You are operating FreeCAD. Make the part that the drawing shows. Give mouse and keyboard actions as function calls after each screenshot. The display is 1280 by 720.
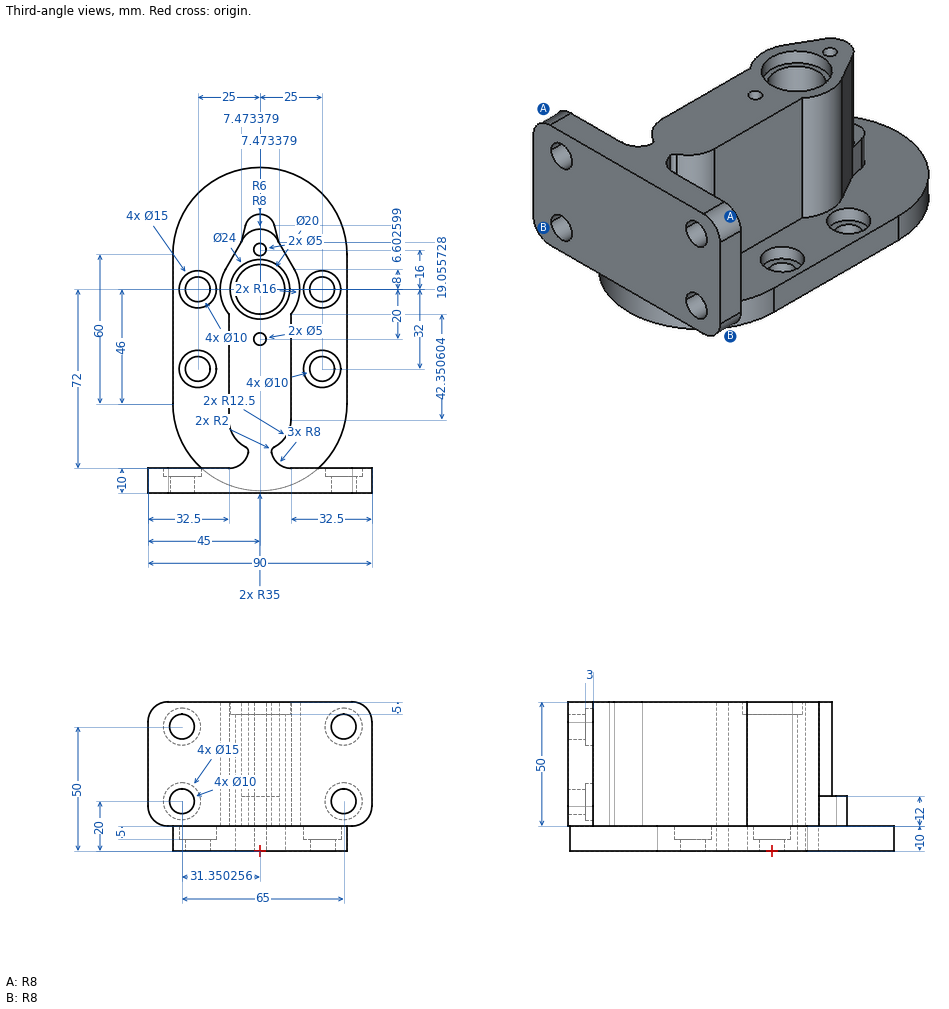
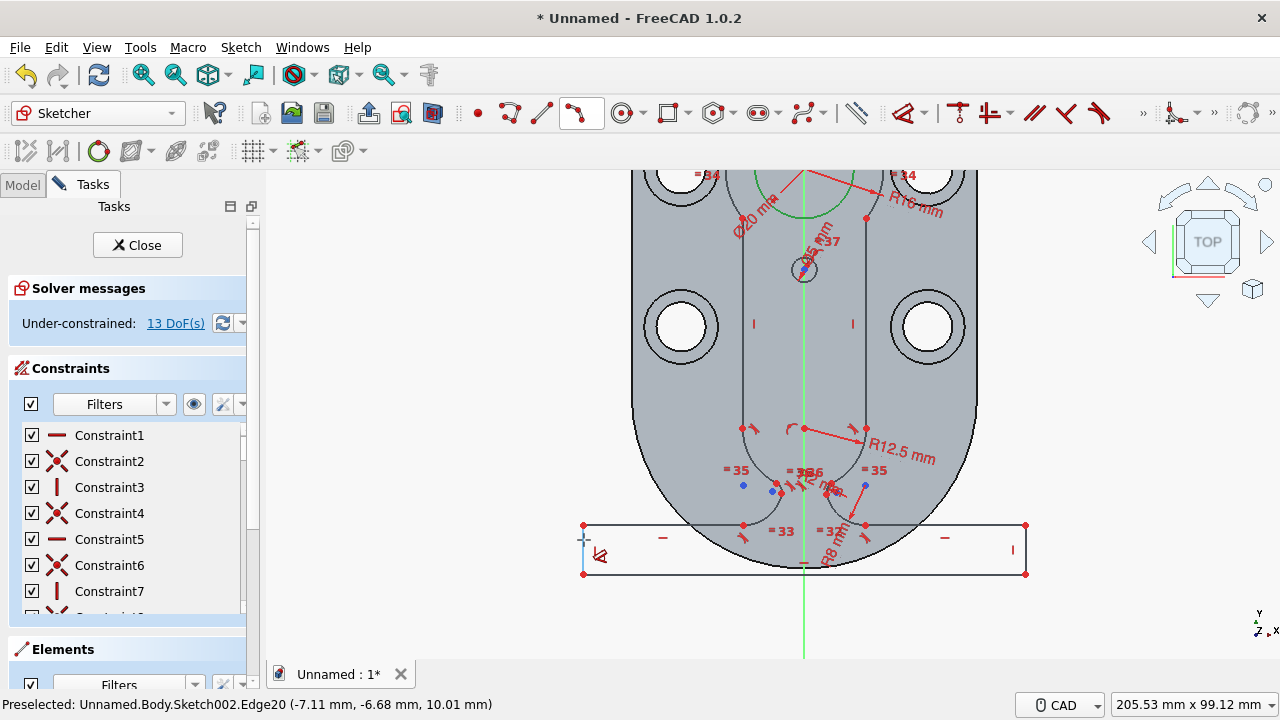
click(583, 540)
click(549, 550)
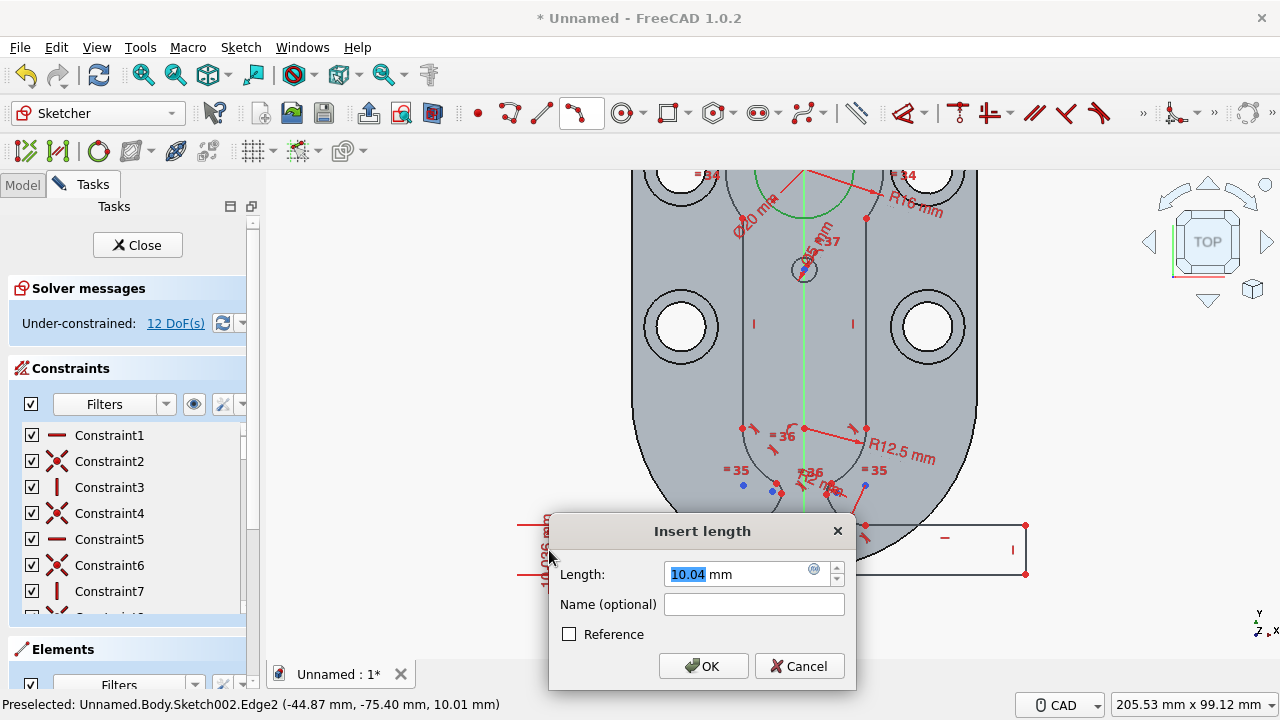
text(10)
key(Return)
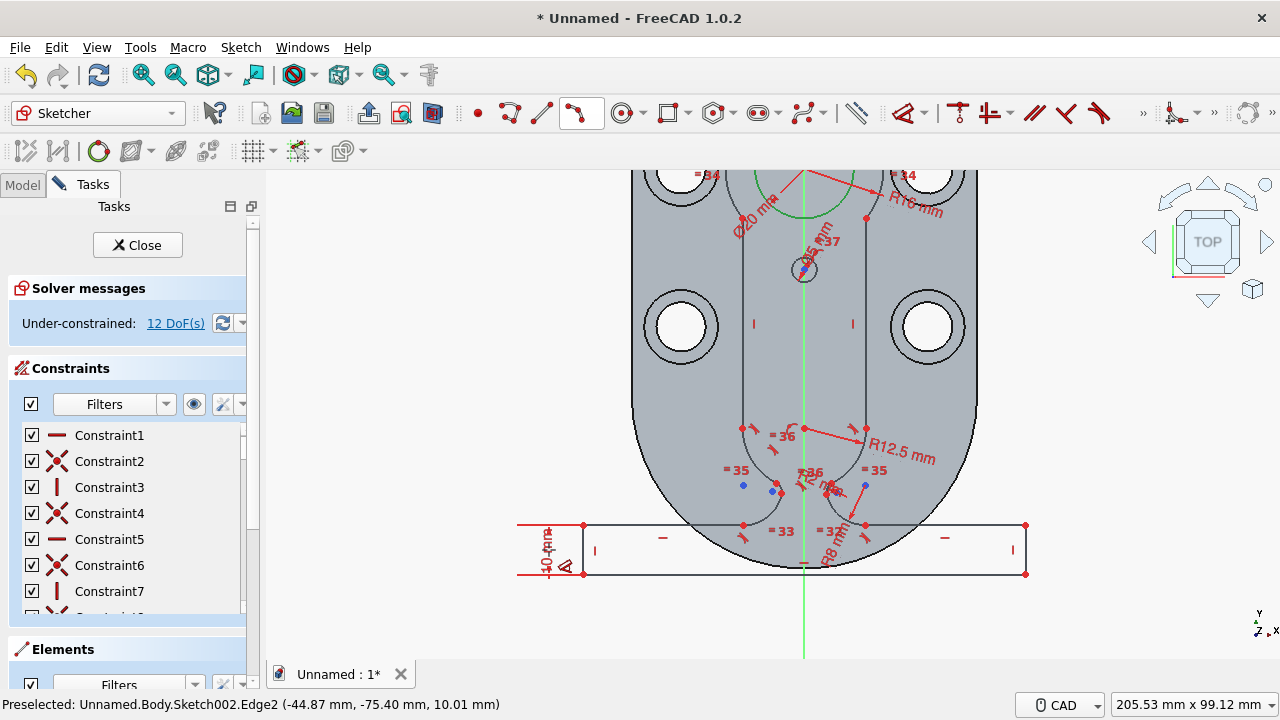
click(716, 575)
click(703, 609)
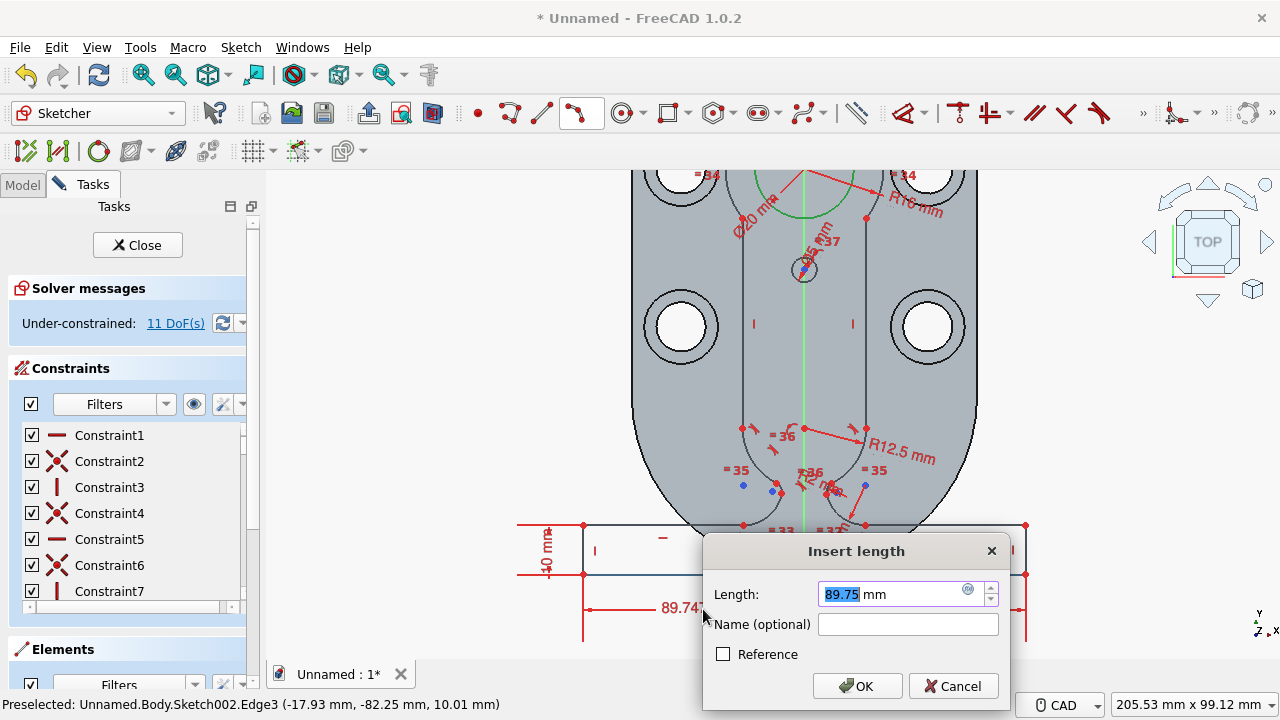
text(90)
key(Return)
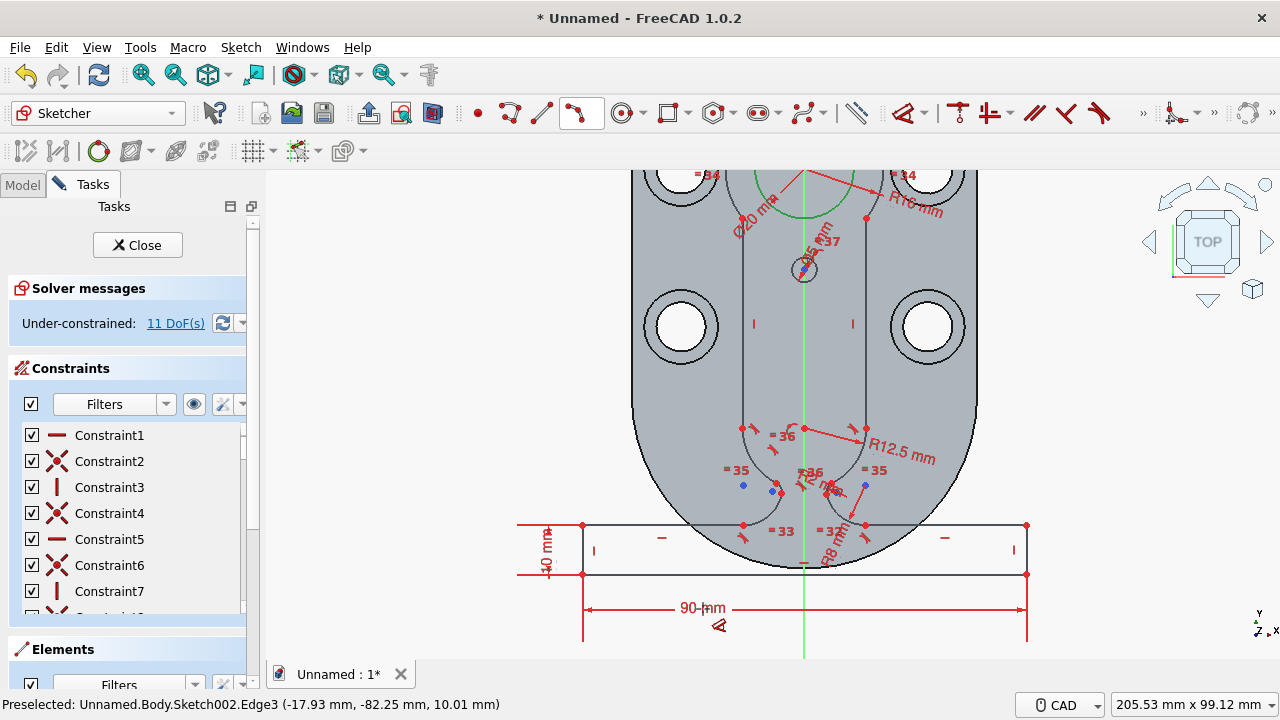
click(1027, 560)
click(1061, 550)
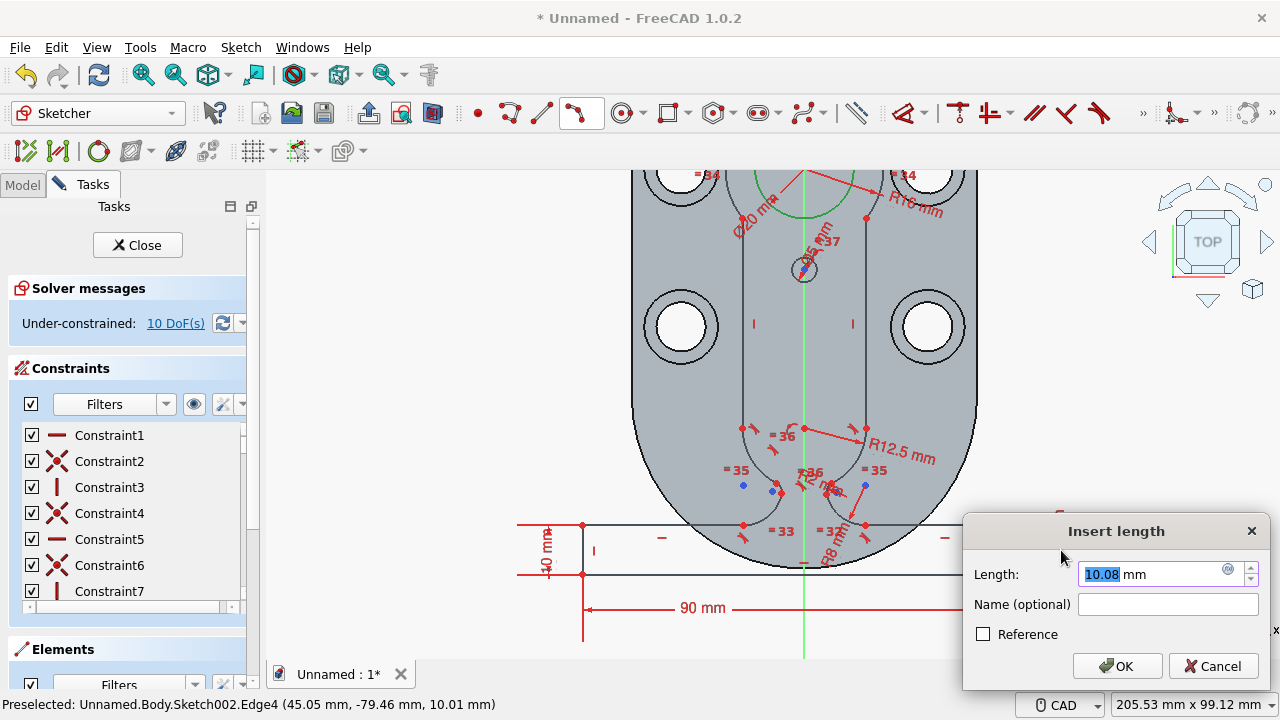
text(10)
key(Return)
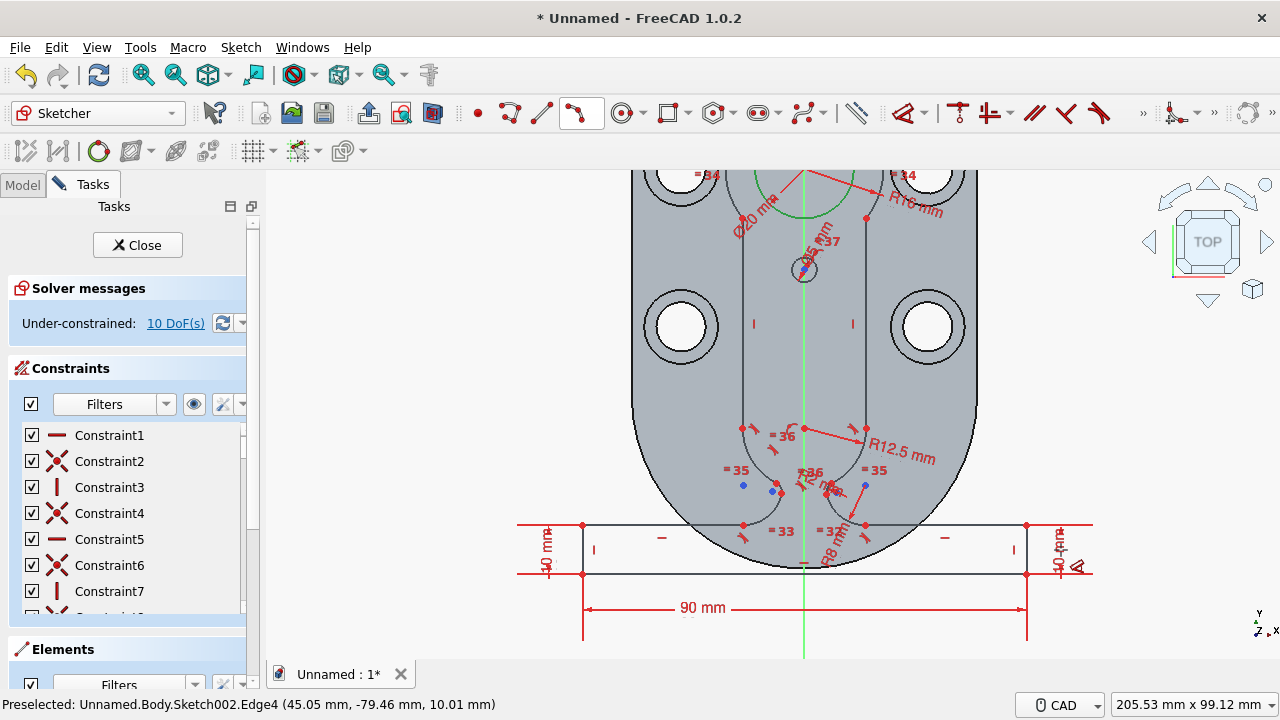
scroll(583, 540, down, 3)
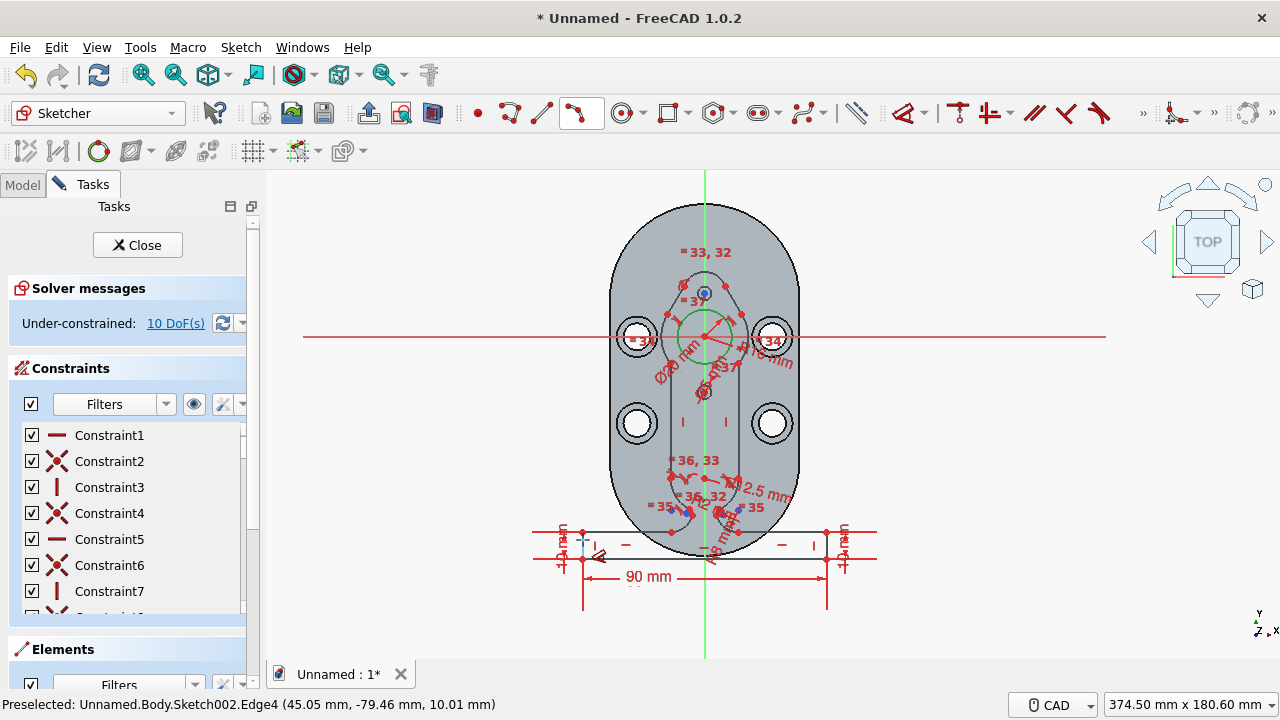
scroll(742, 315, up, 4)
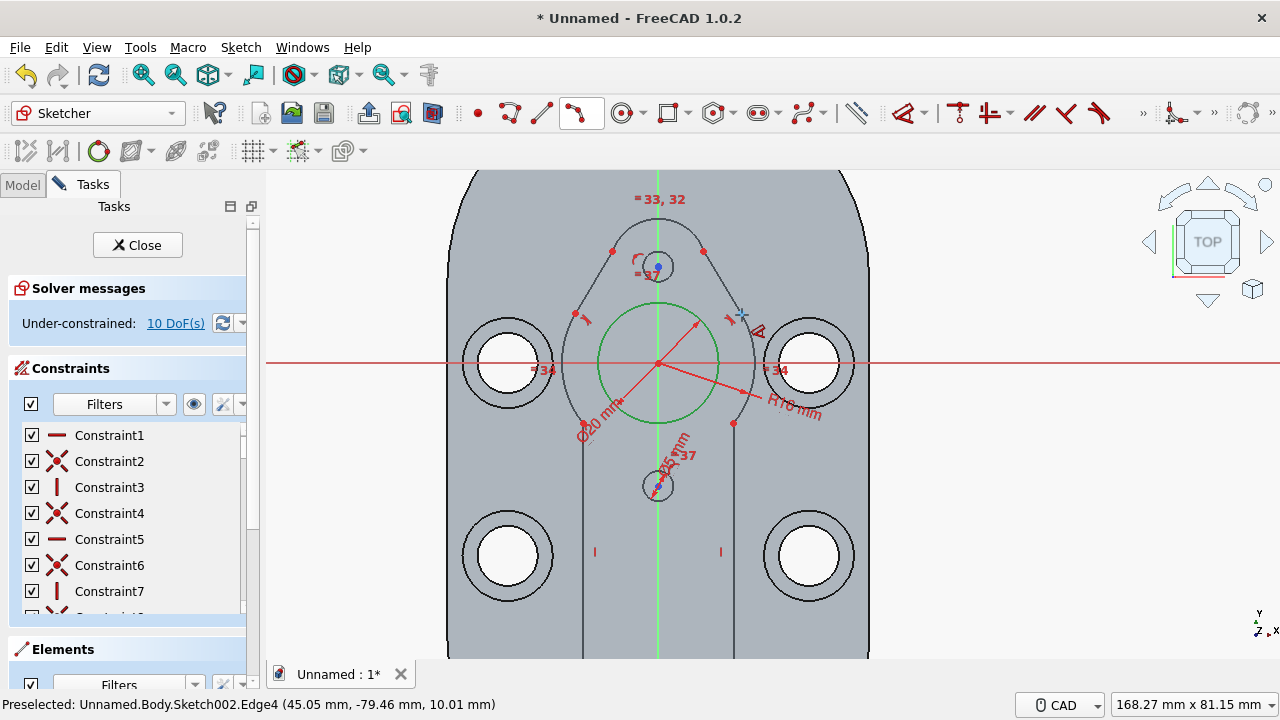
click(741, 314)
click(775, 338)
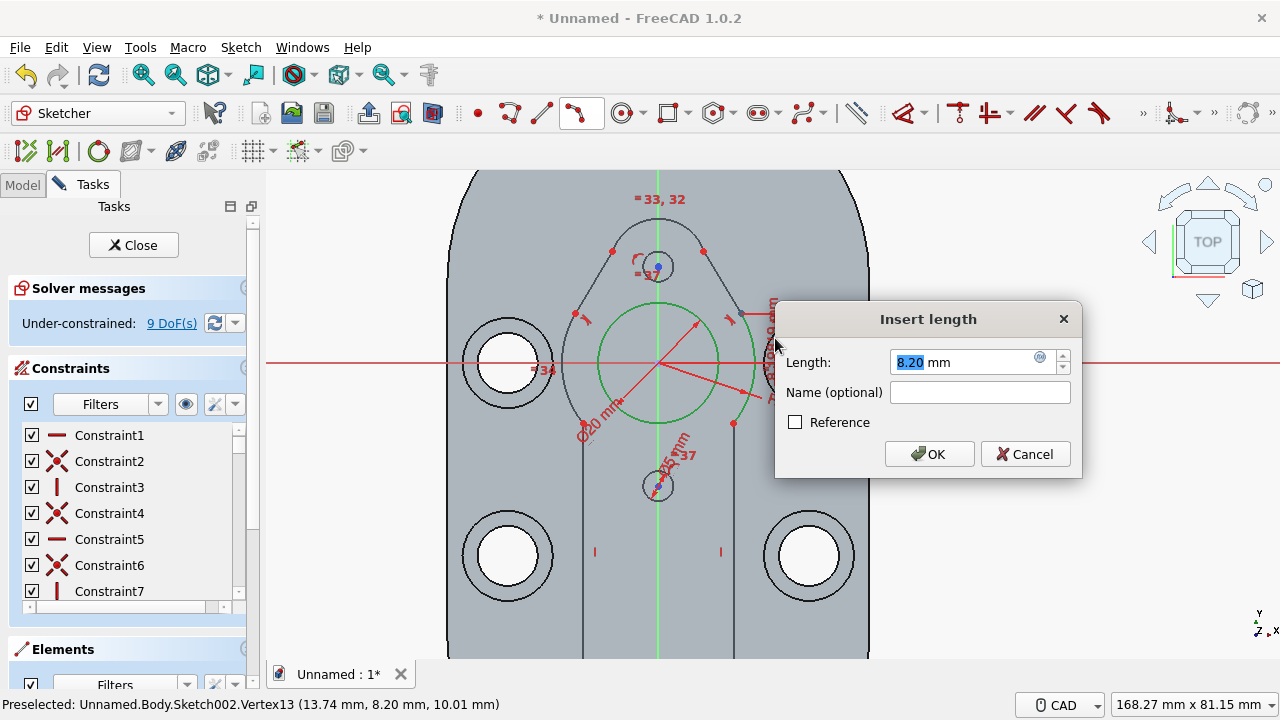
text(8)
key(Return)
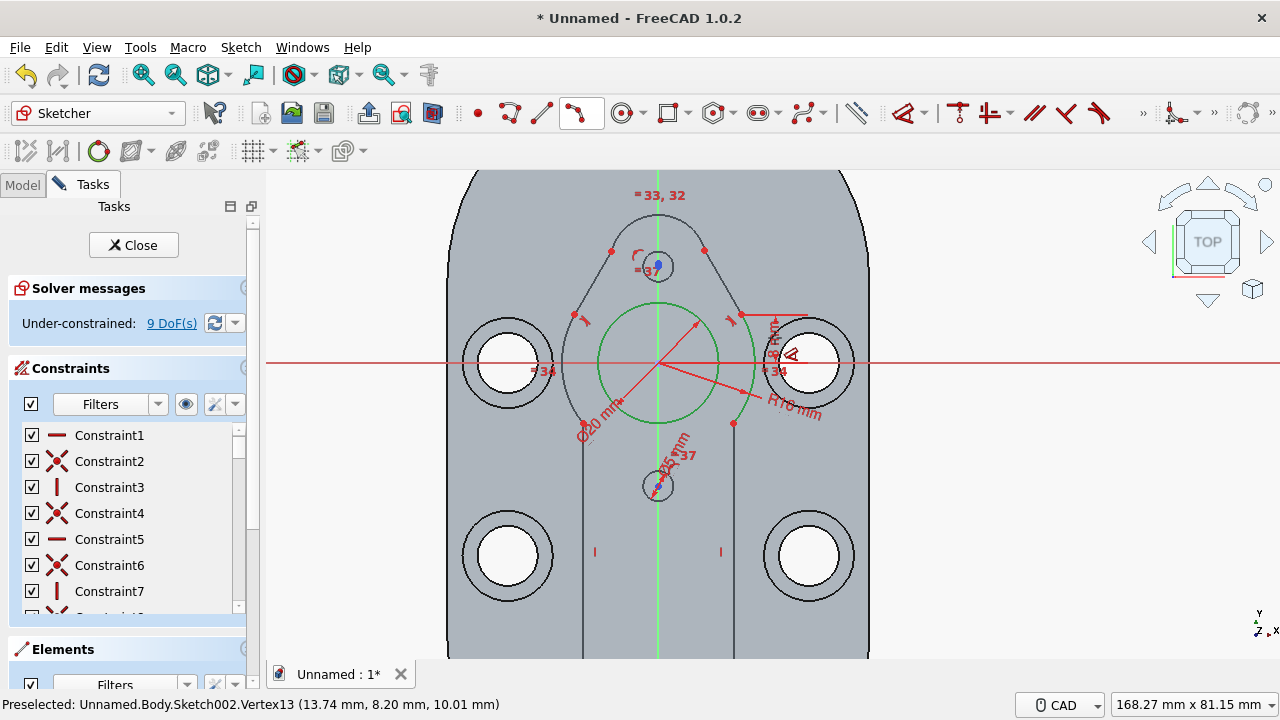
click(575, 315)
click(541, 339)